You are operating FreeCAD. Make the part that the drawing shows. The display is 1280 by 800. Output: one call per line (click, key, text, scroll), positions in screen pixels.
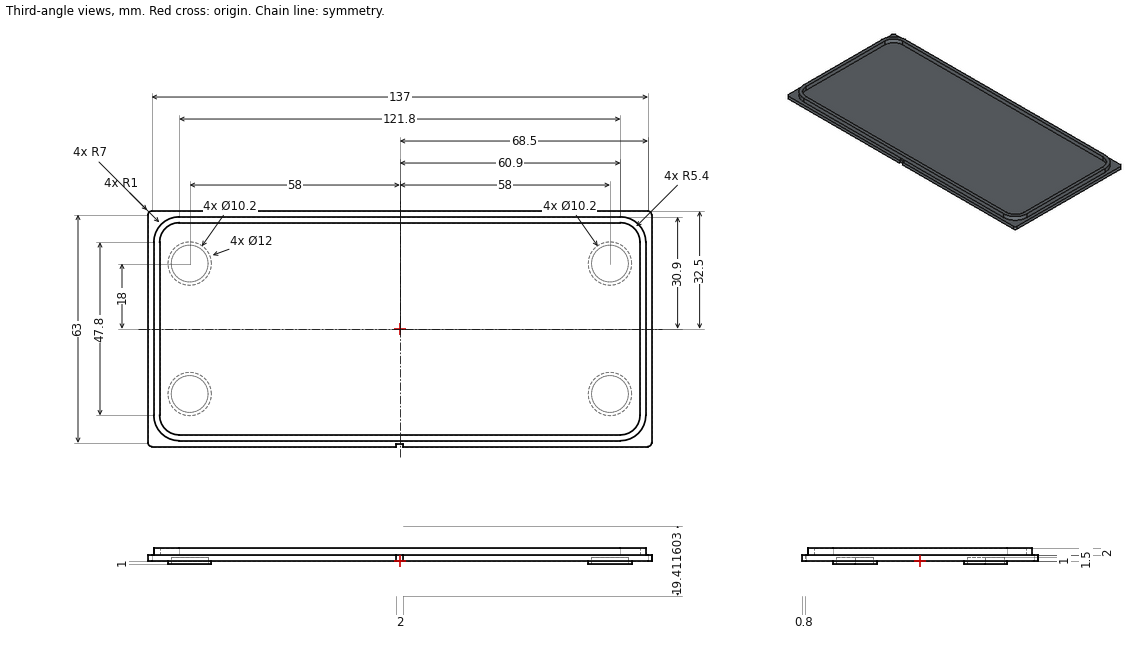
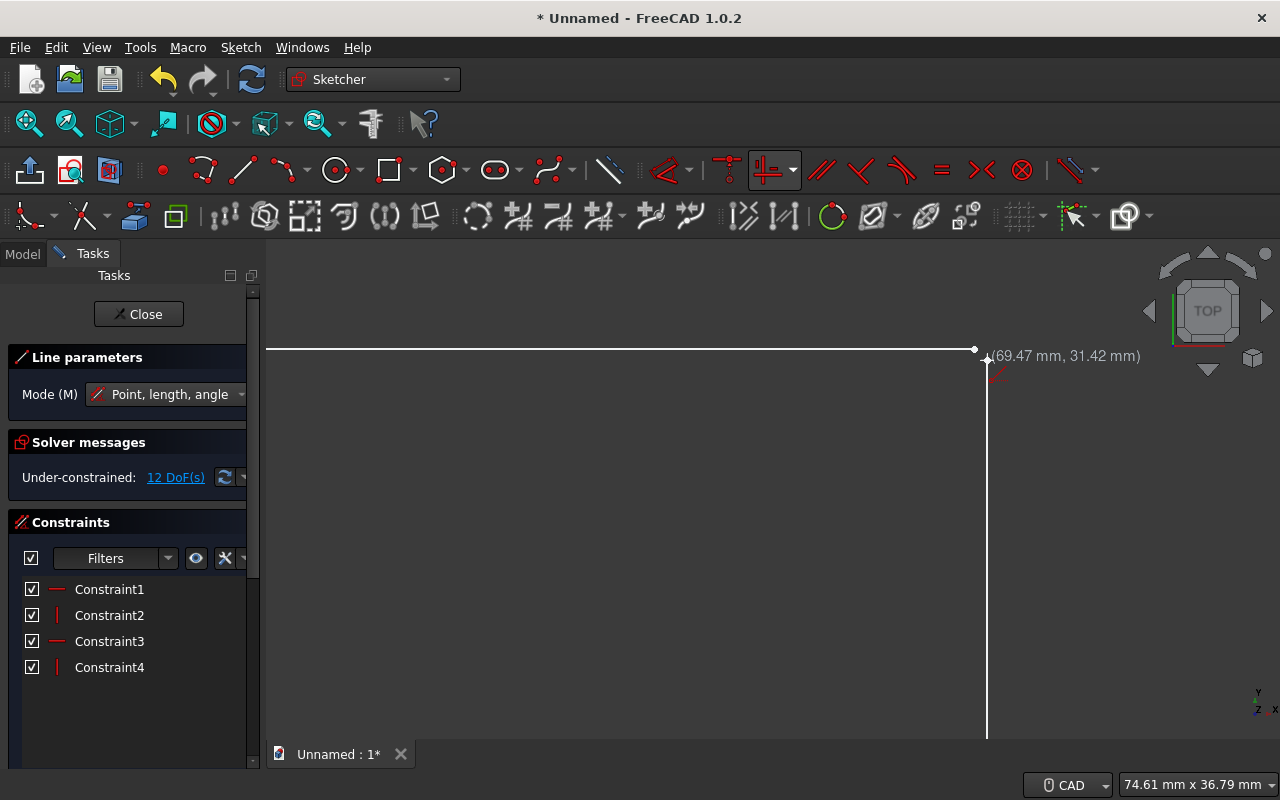
click(284, 170)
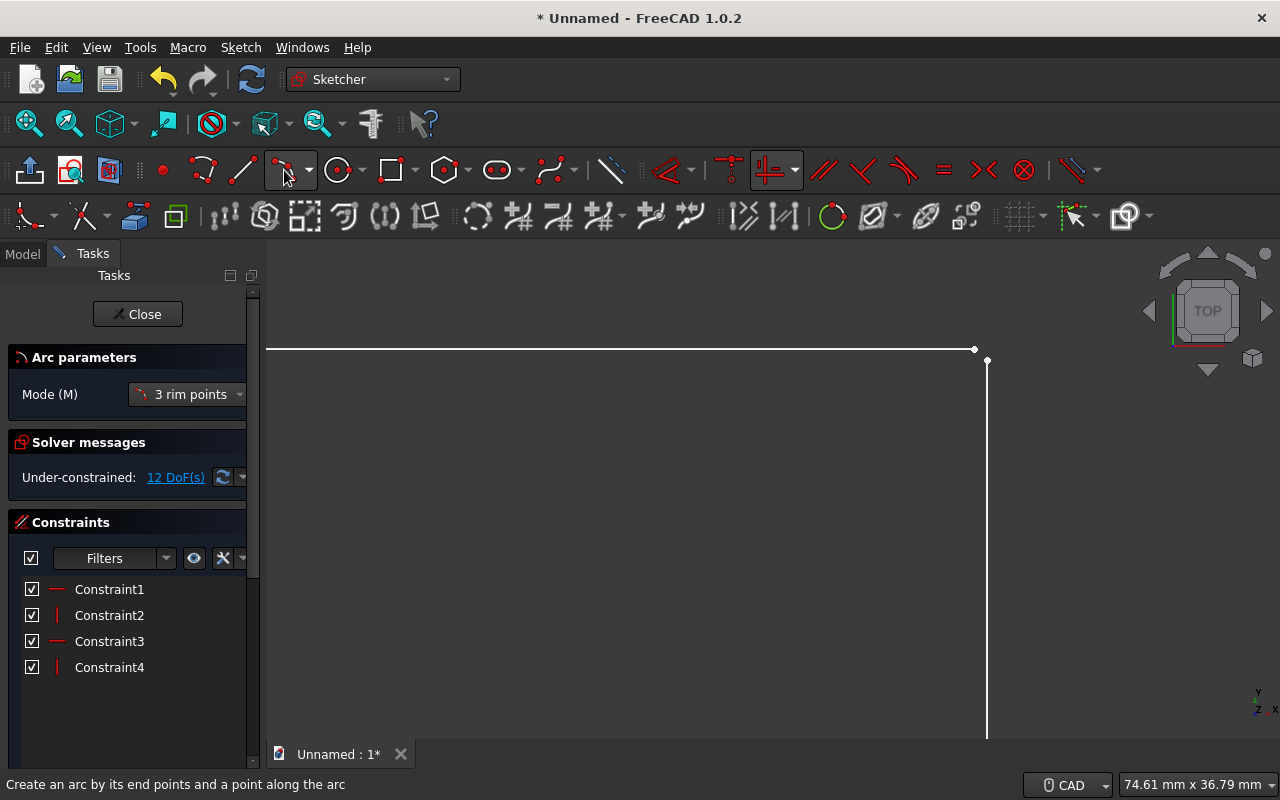
scroll(990, 360, down, 6)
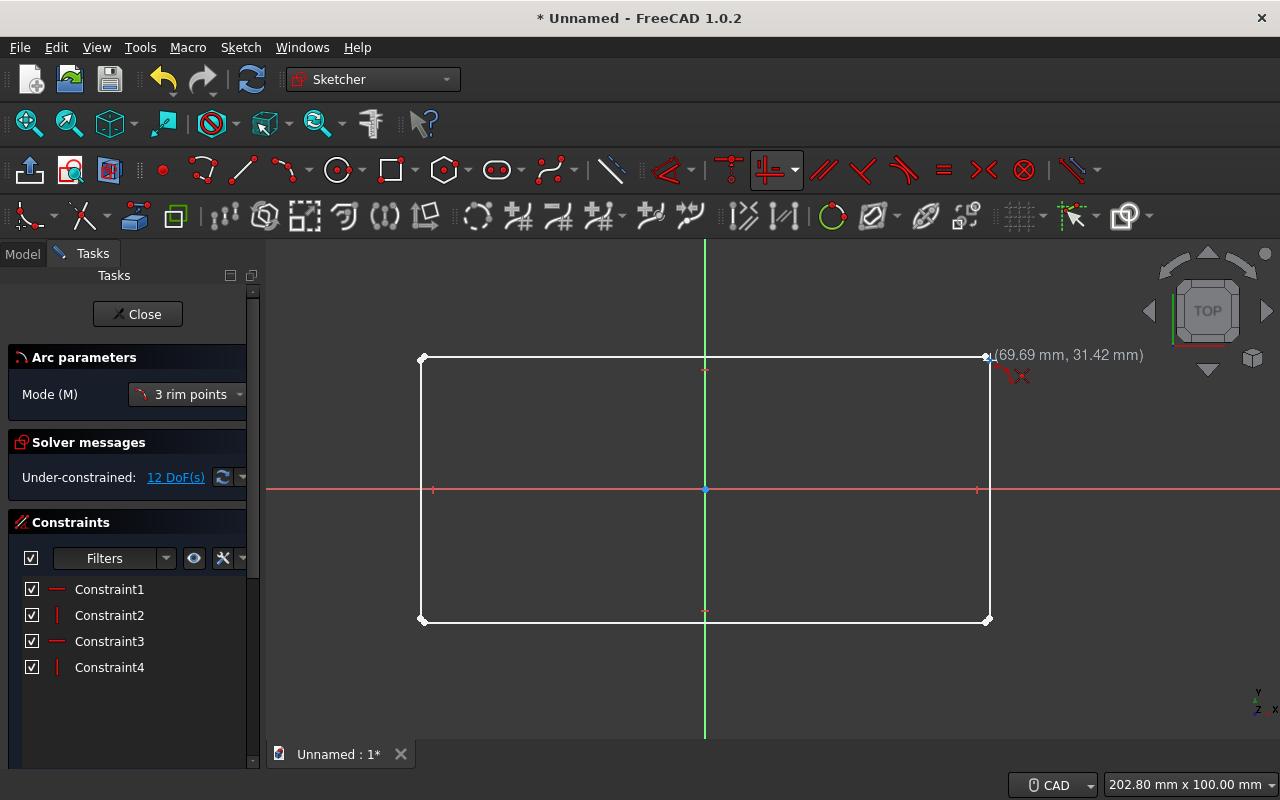
scroll(425, 356, up, 6)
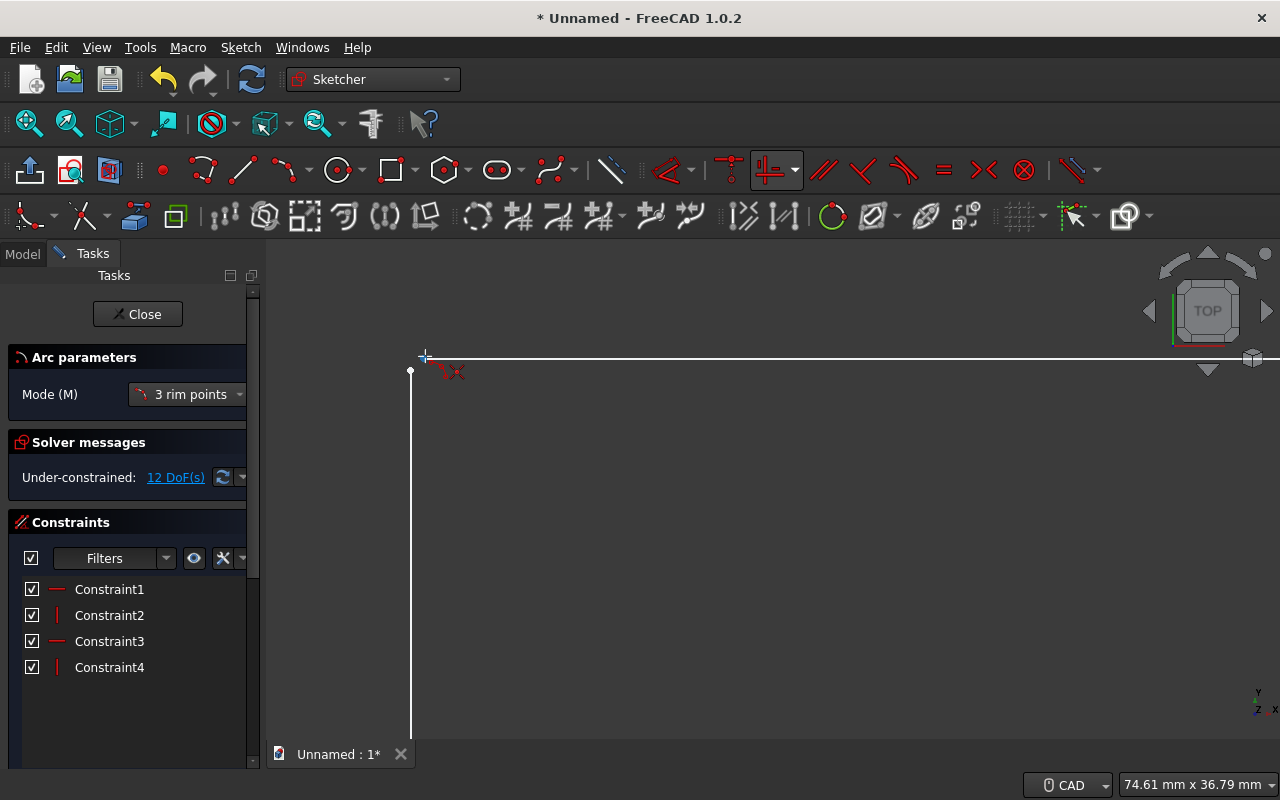
click(424, 359)
click(411, 370)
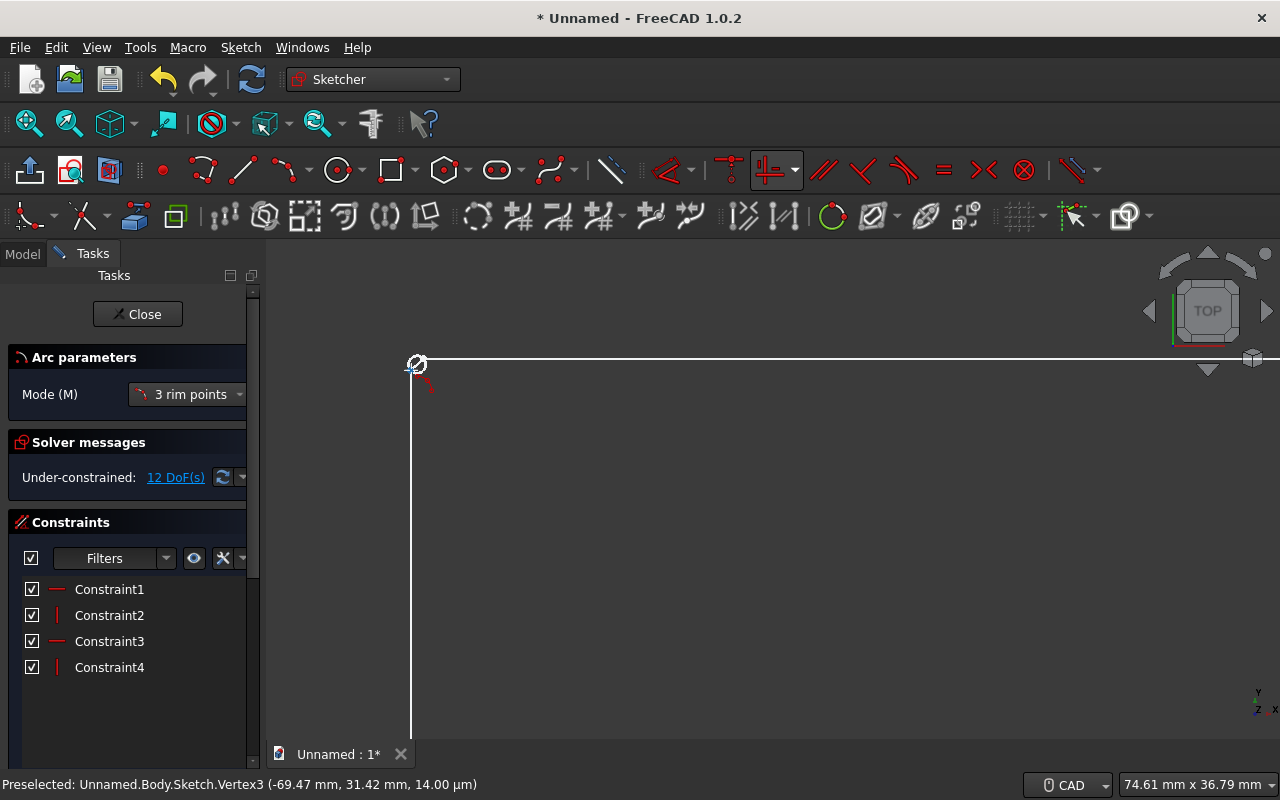
scroll(414, 360, up, 7)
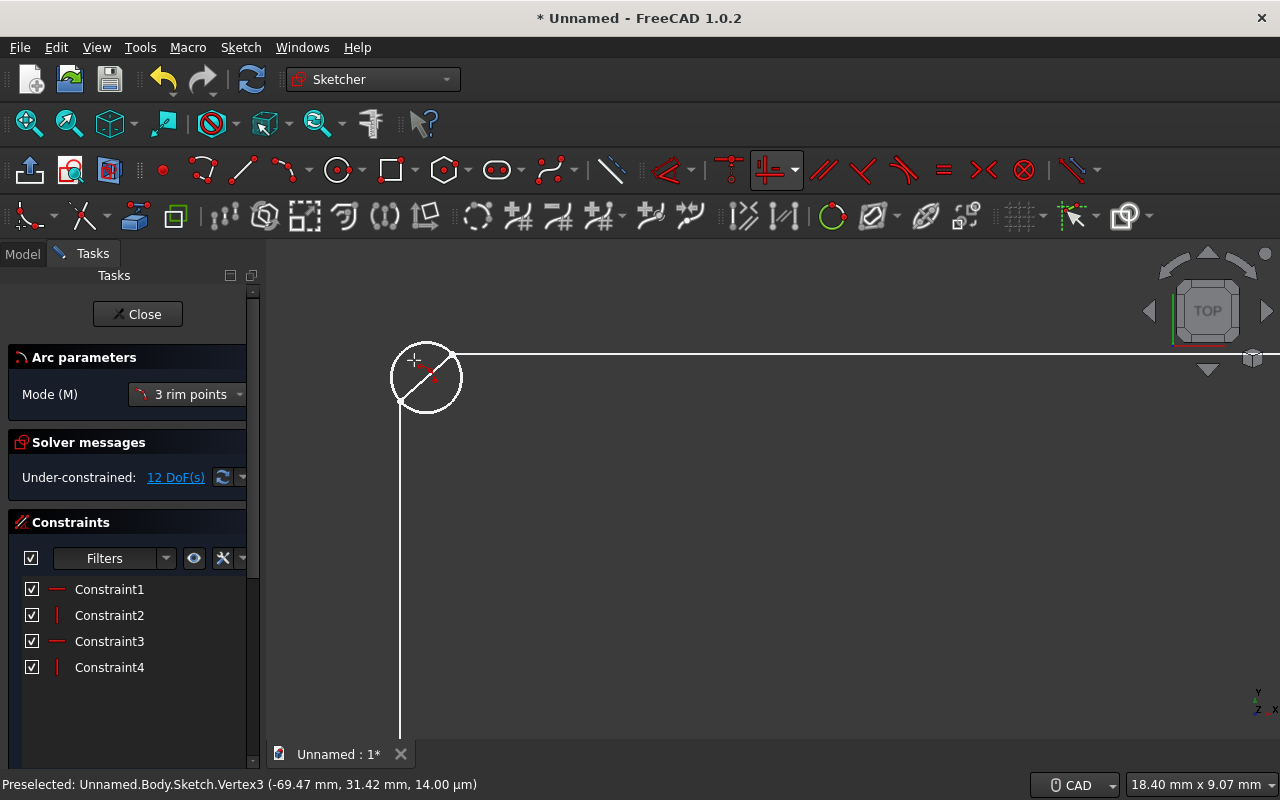
click(415, 358)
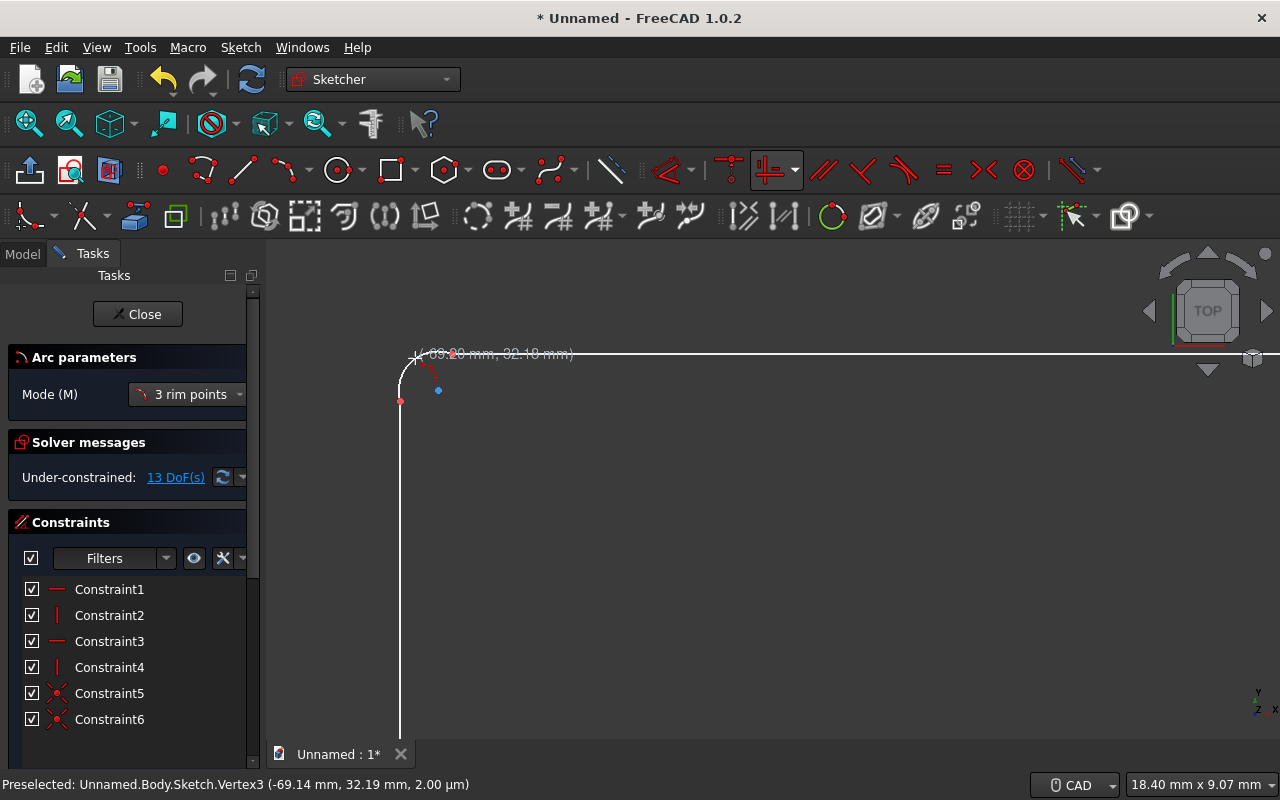
scroll(422, 357, down, 13)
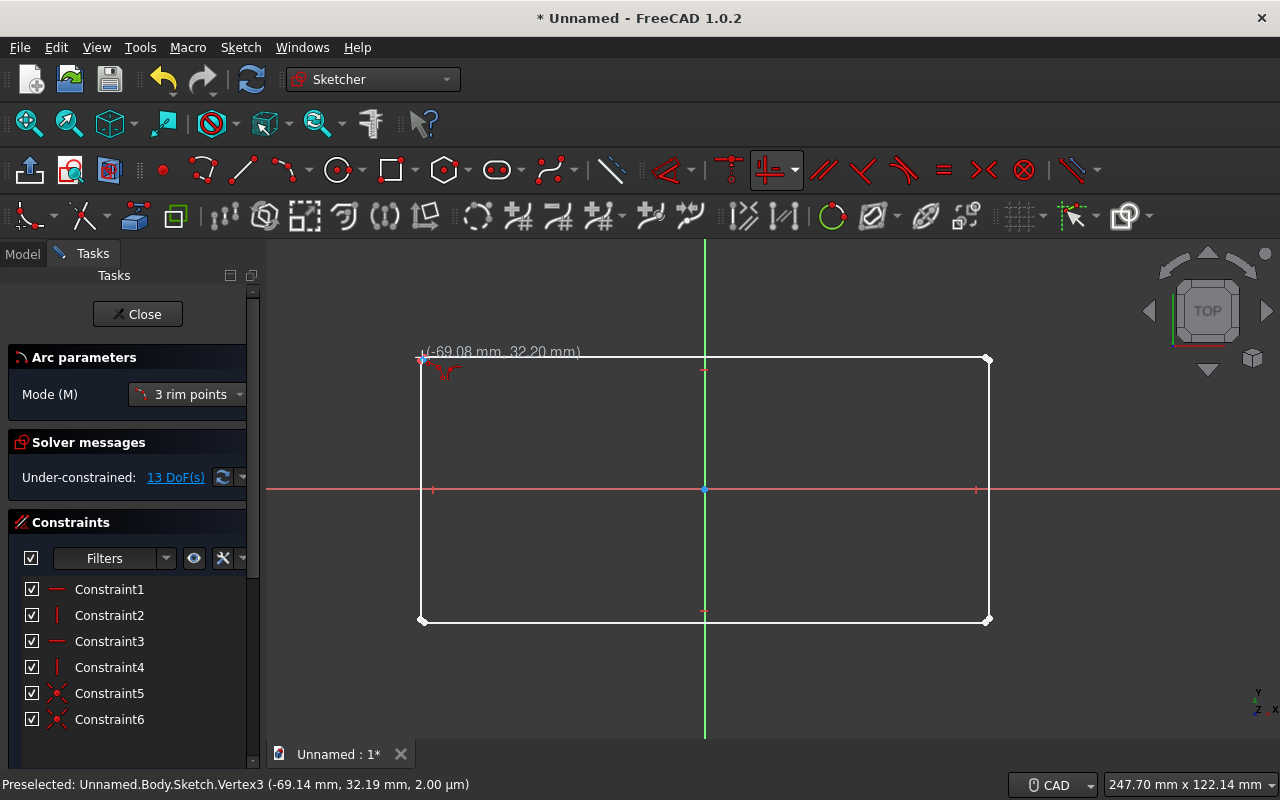
scroll(420, 618, up, 6)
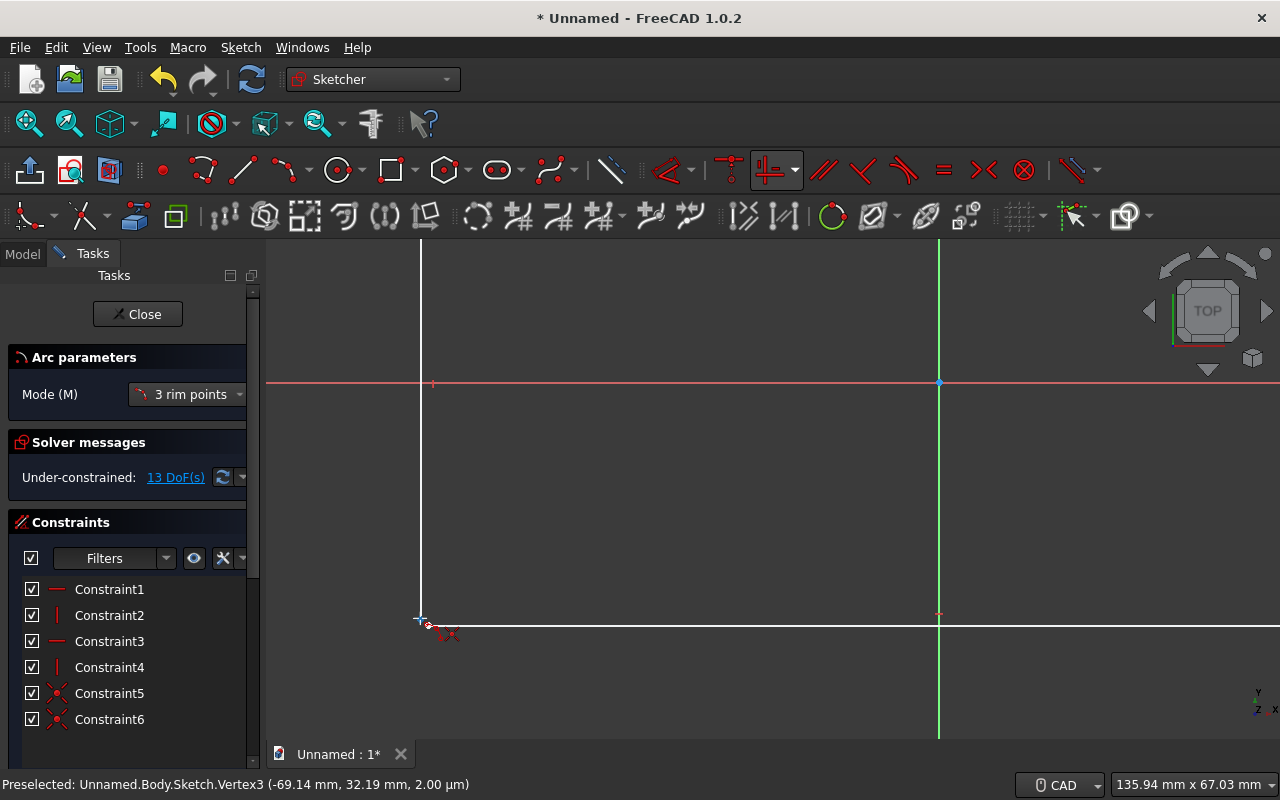
click(421, 620)
click(435, 631)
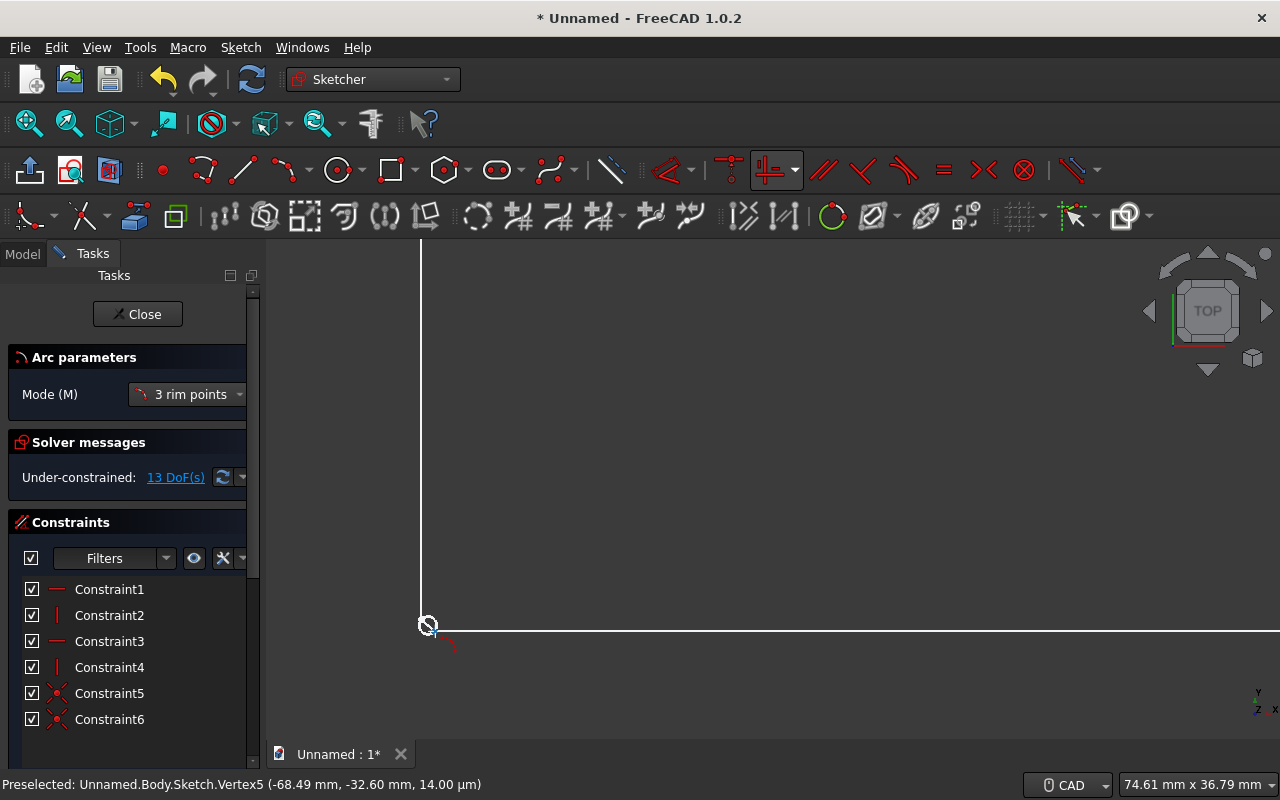
scroll(425, 626, up, 7)